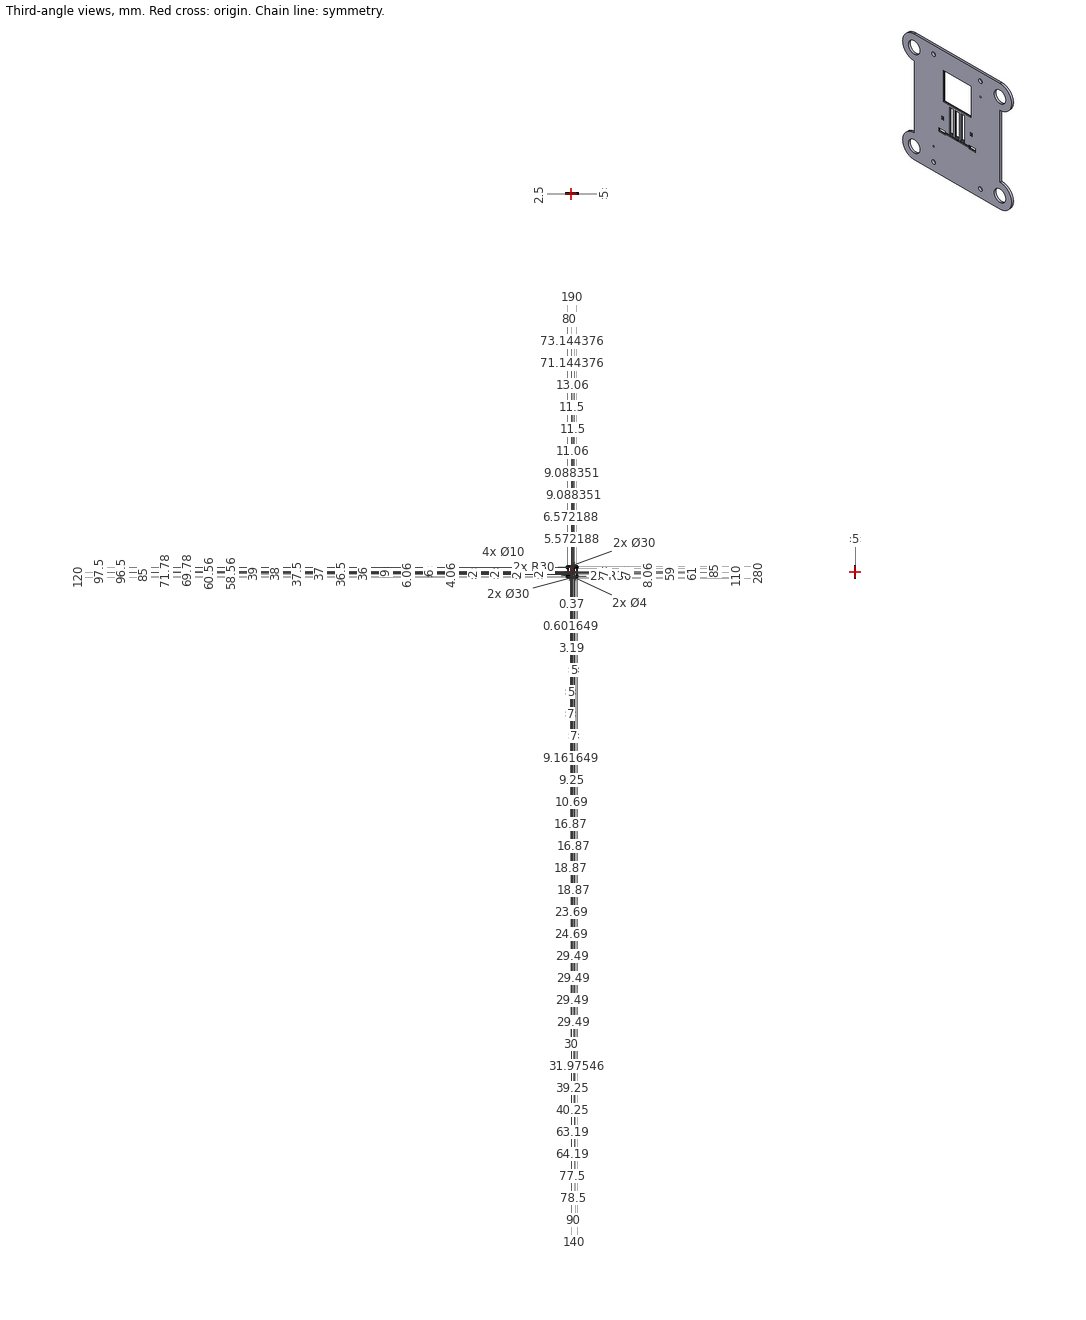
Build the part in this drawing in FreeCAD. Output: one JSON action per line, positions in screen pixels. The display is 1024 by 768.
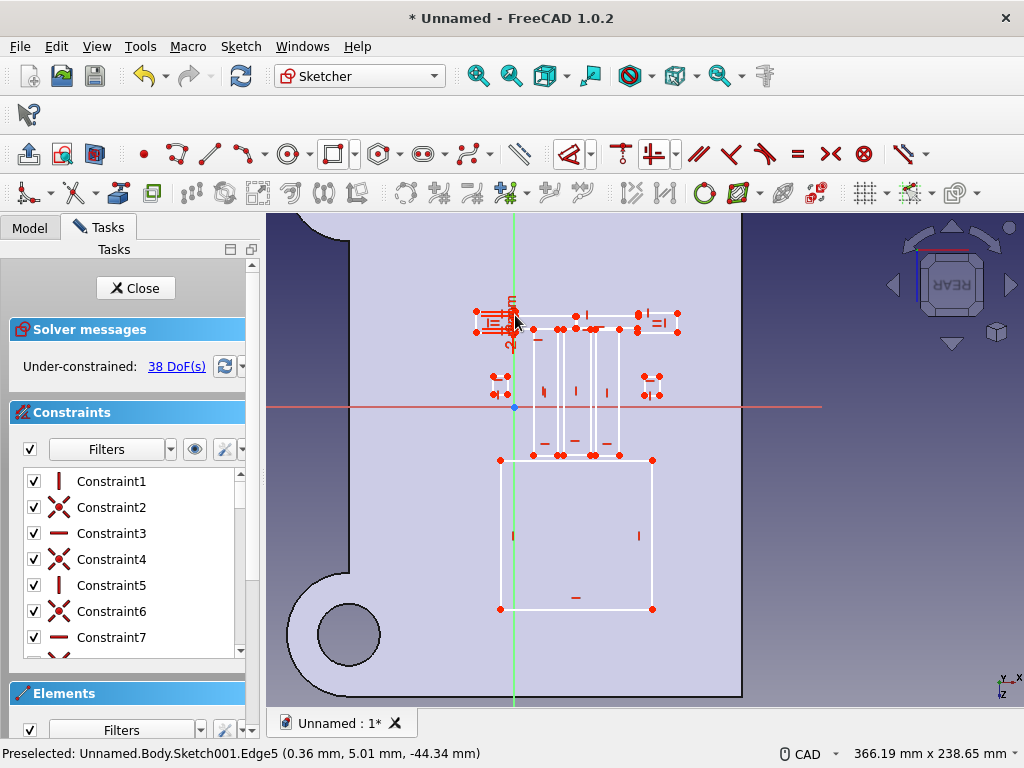
{"action": "scroll", "coordinate": [493, 382], "scroll_direction": "up", "scroll_amount": 5}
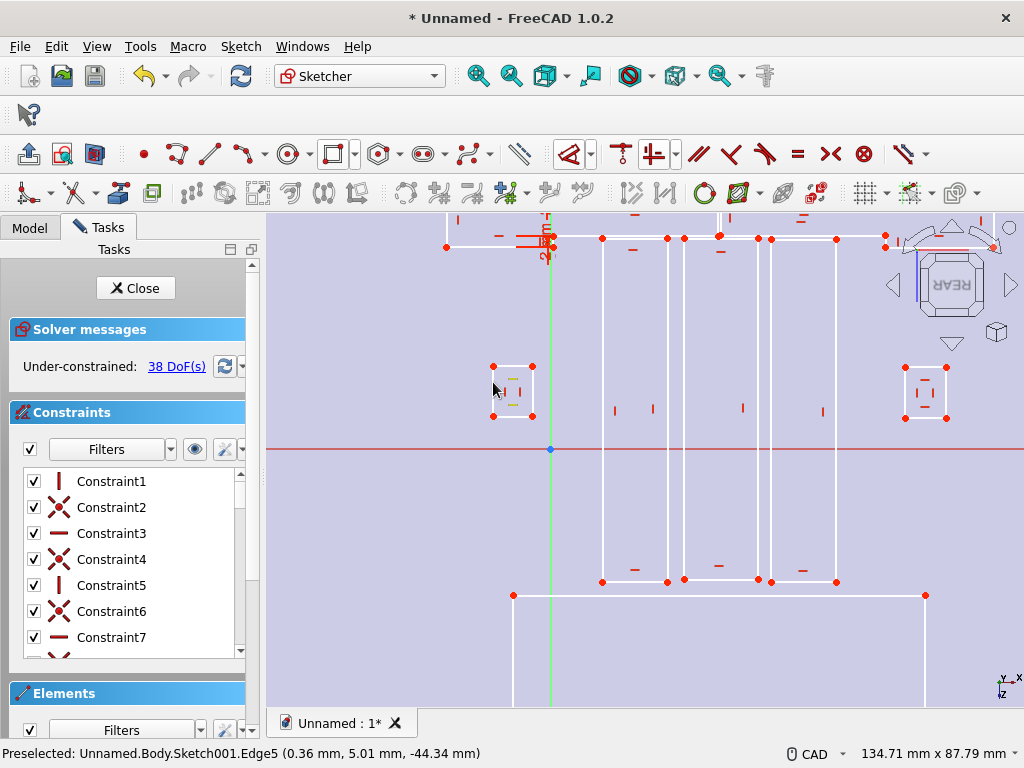
{"action": "left_click", "coordinate": [493, 381]}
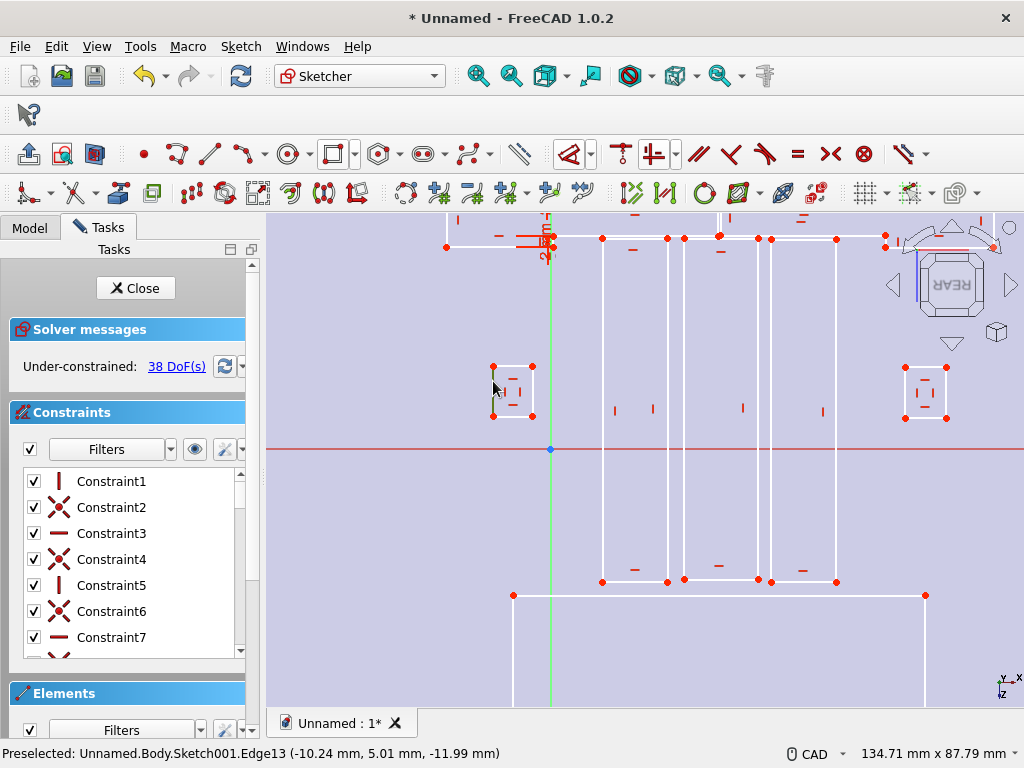
{"action": "left_click", "coordinate": [590, 154]}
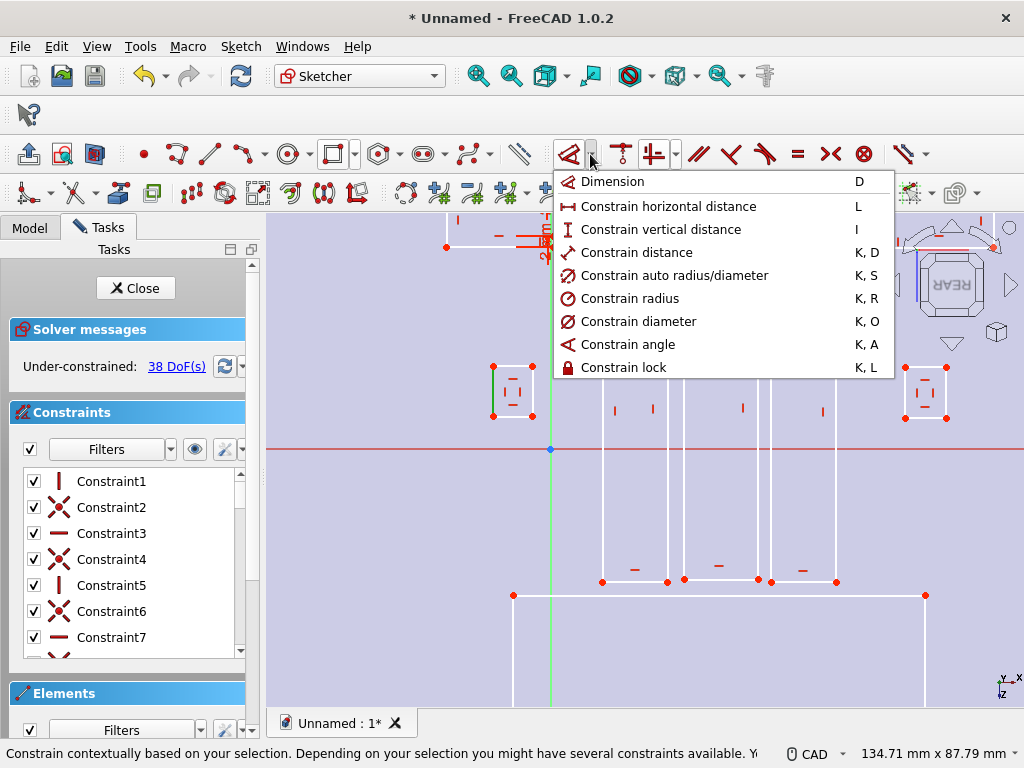
{"action": "left_click", "coordinate": [724, 230]}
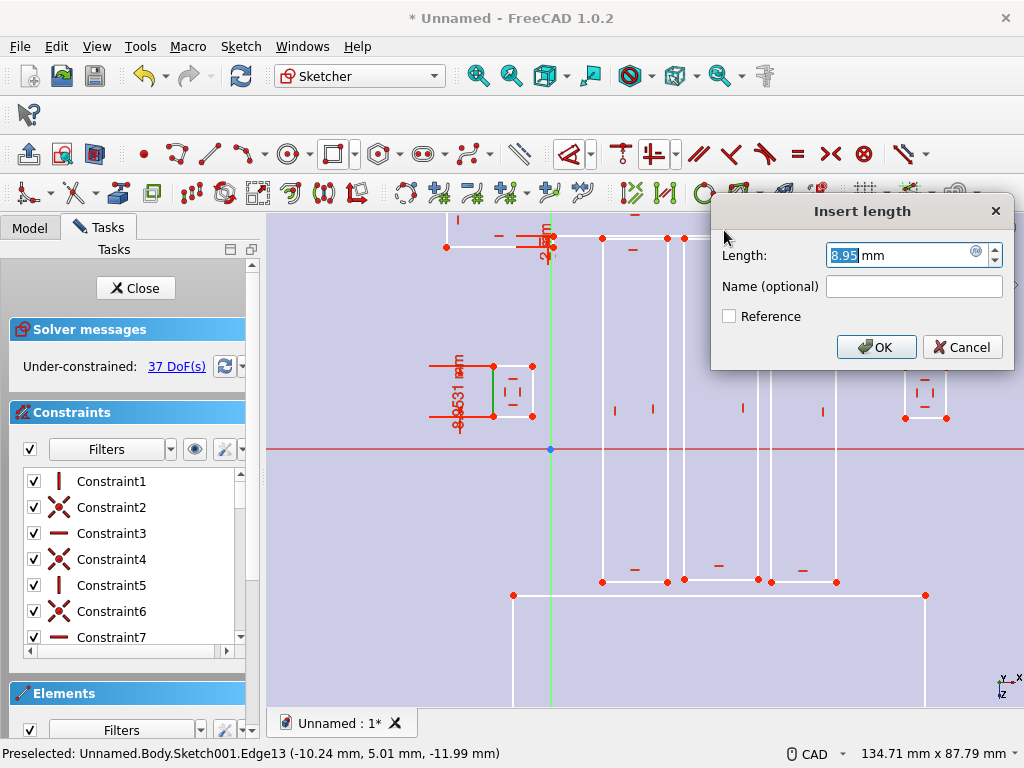
{"action": "type", "text": "9"}
{"action": "key", "text": "Return"}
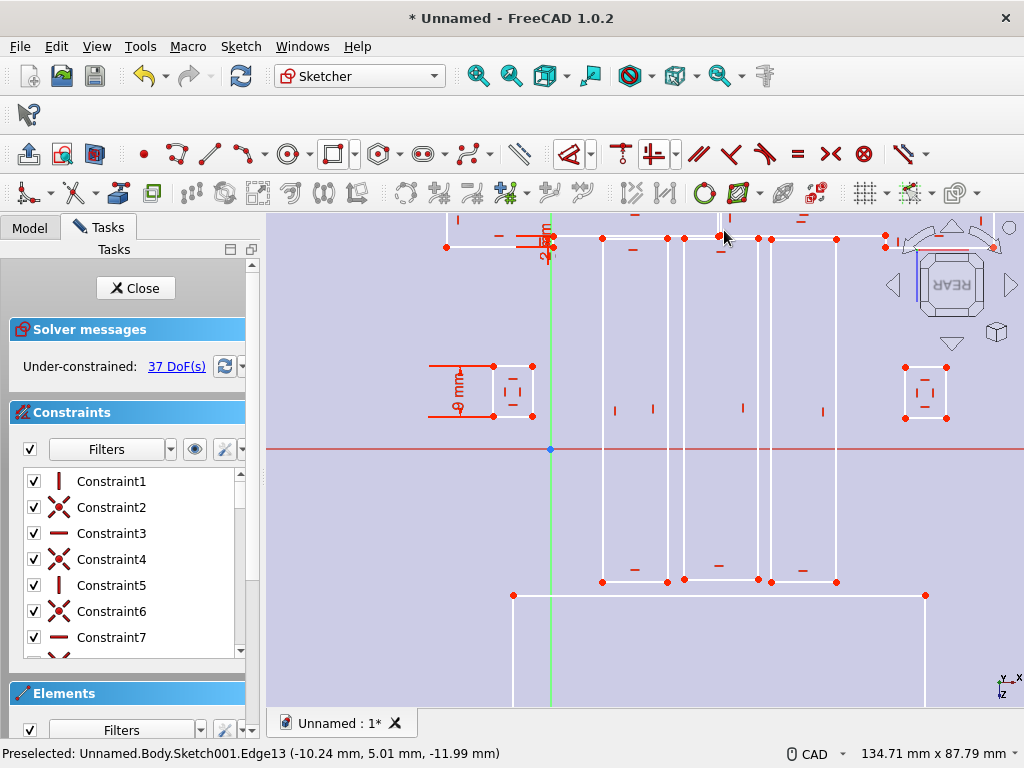
{"action": "left_click", "coordinate": [505, 417]}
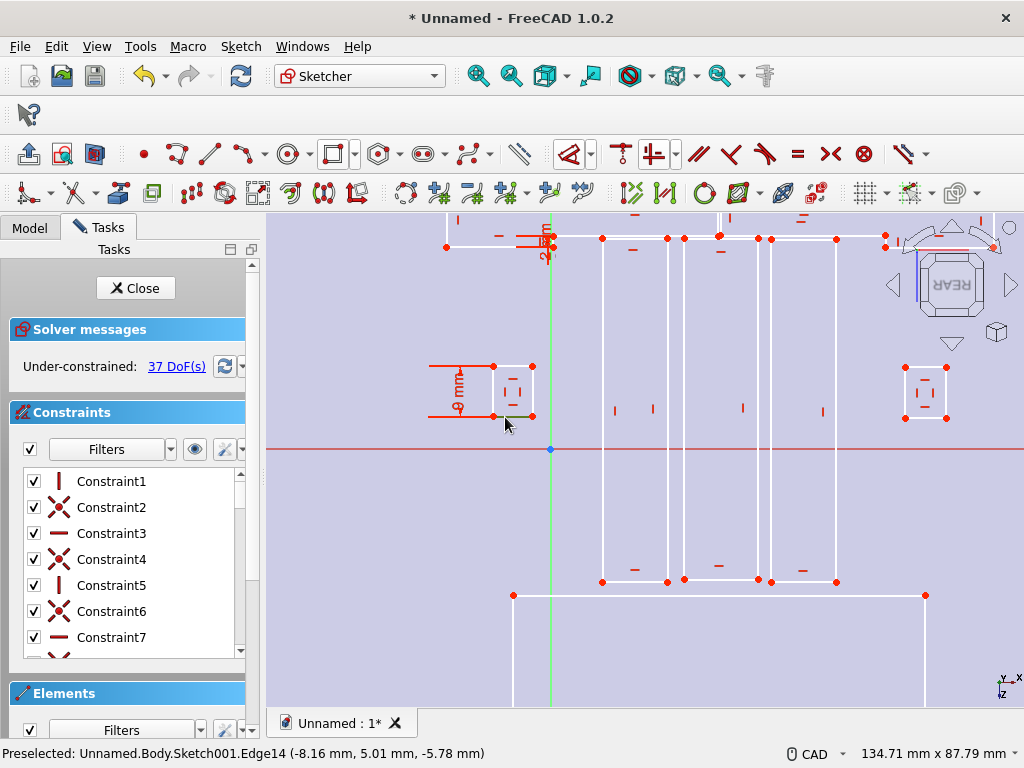
{"action": "left_click", "coordinate": [590, 154]}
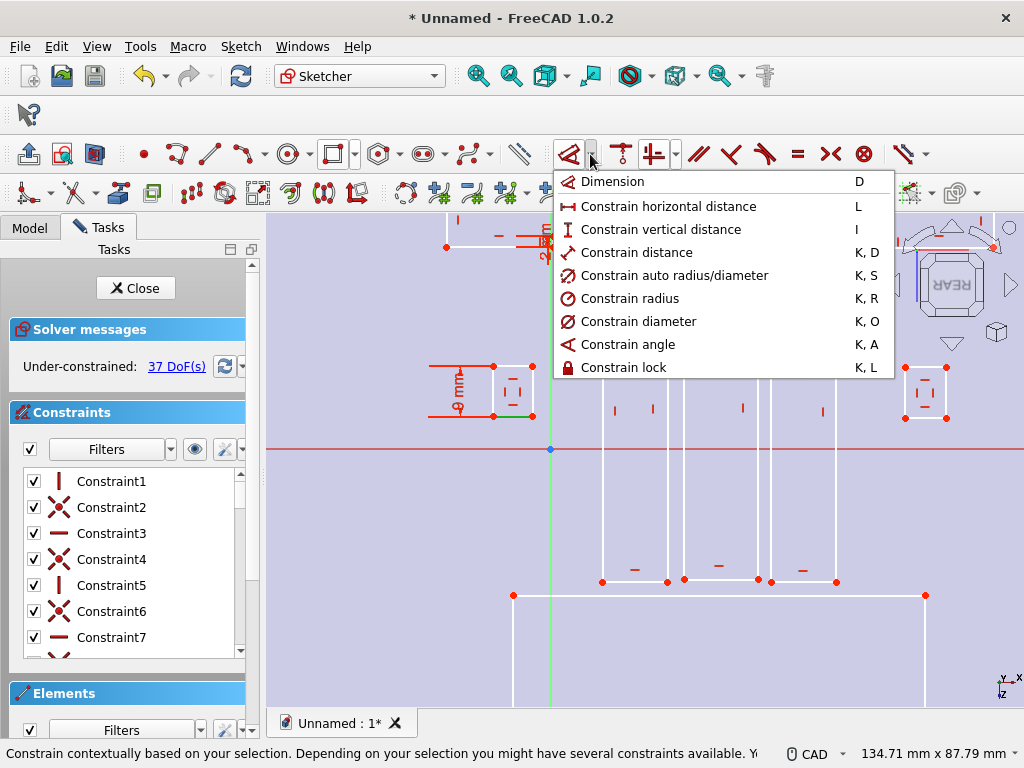
{"action": "left_click", "coordinate": [724, 206]}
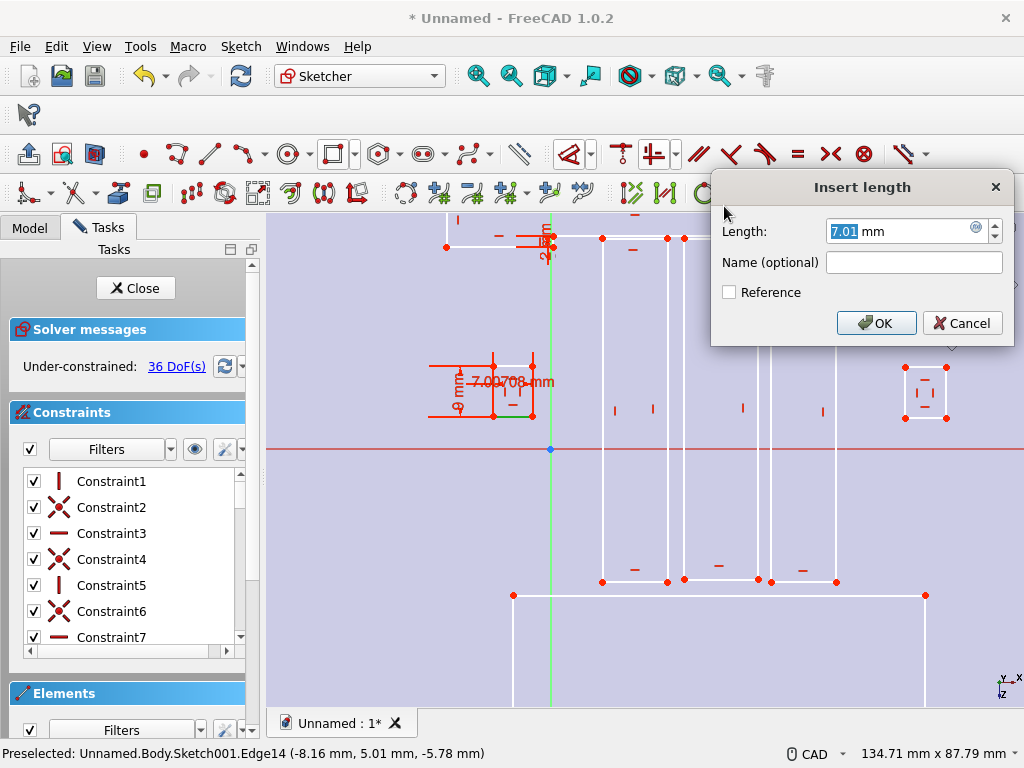
{"action": "type", "text": "7"}
{"action": "key", "text": "Return"}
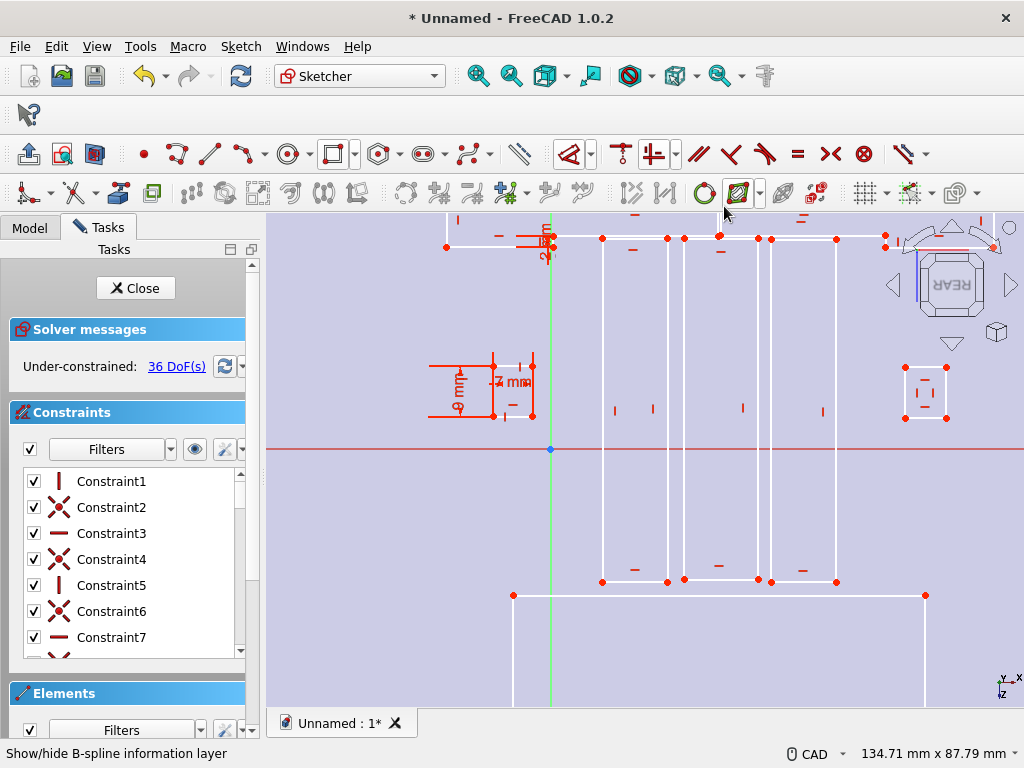
{"action": "scroll", "coordinate": [493, 382], "scroll_direction": "down", "scroll_amount": 5}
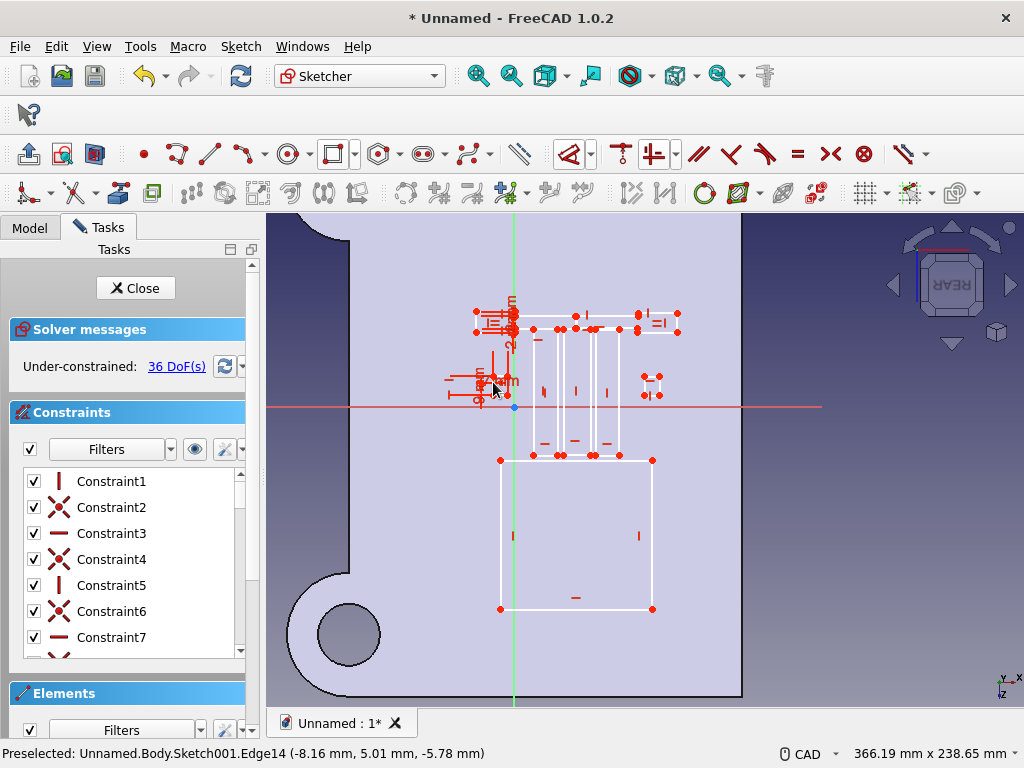
{"action": "scroll", "coordinate": [645, 382], "scroll_direction": "up", "scroll_amount": 5}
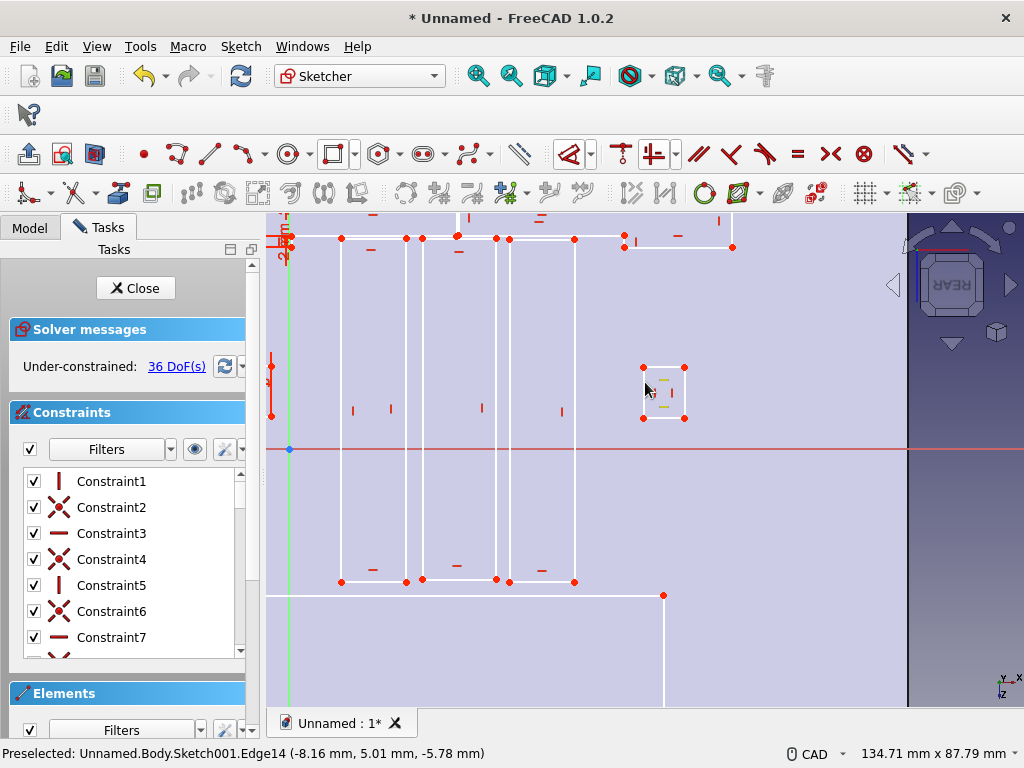
{"action": "left_click", "coordinate": [644, 383]}